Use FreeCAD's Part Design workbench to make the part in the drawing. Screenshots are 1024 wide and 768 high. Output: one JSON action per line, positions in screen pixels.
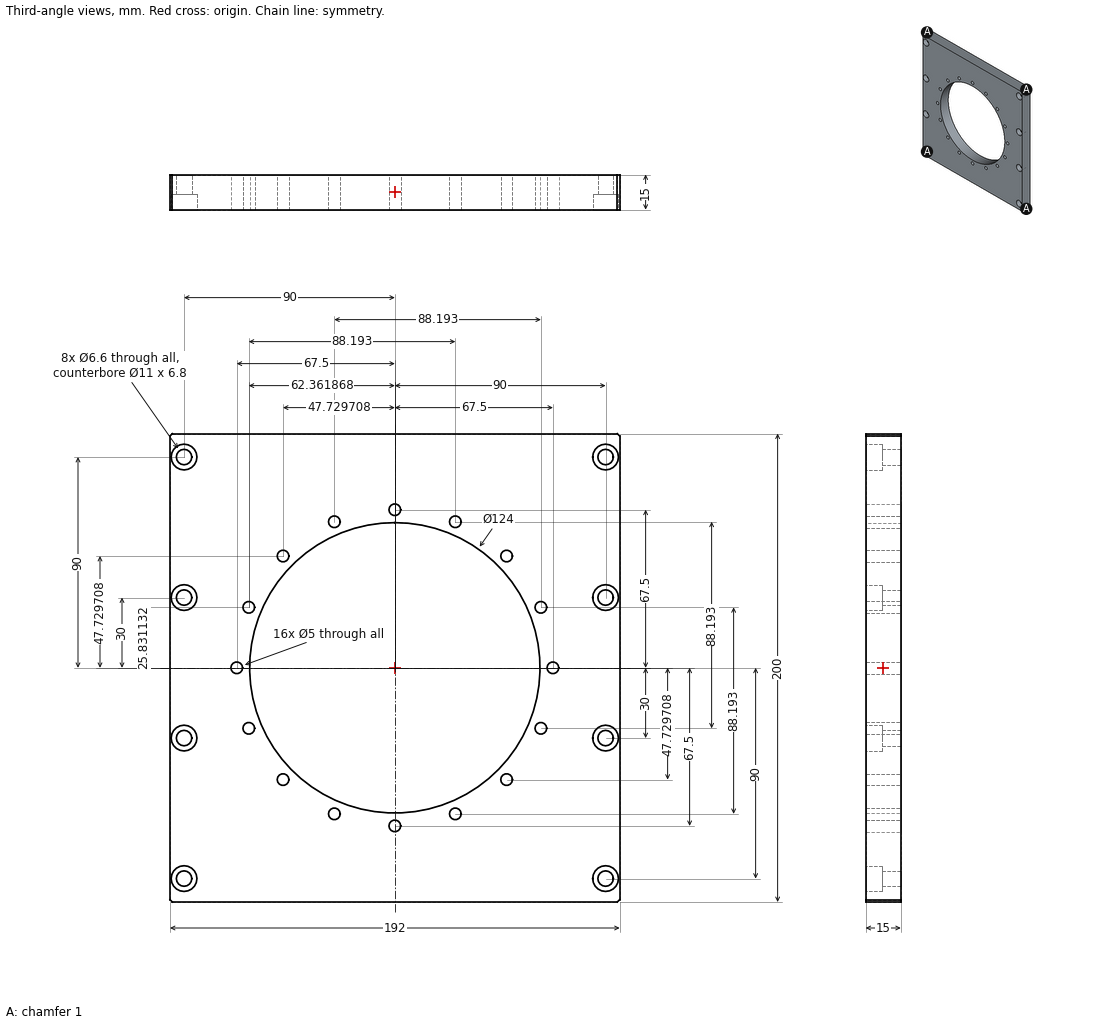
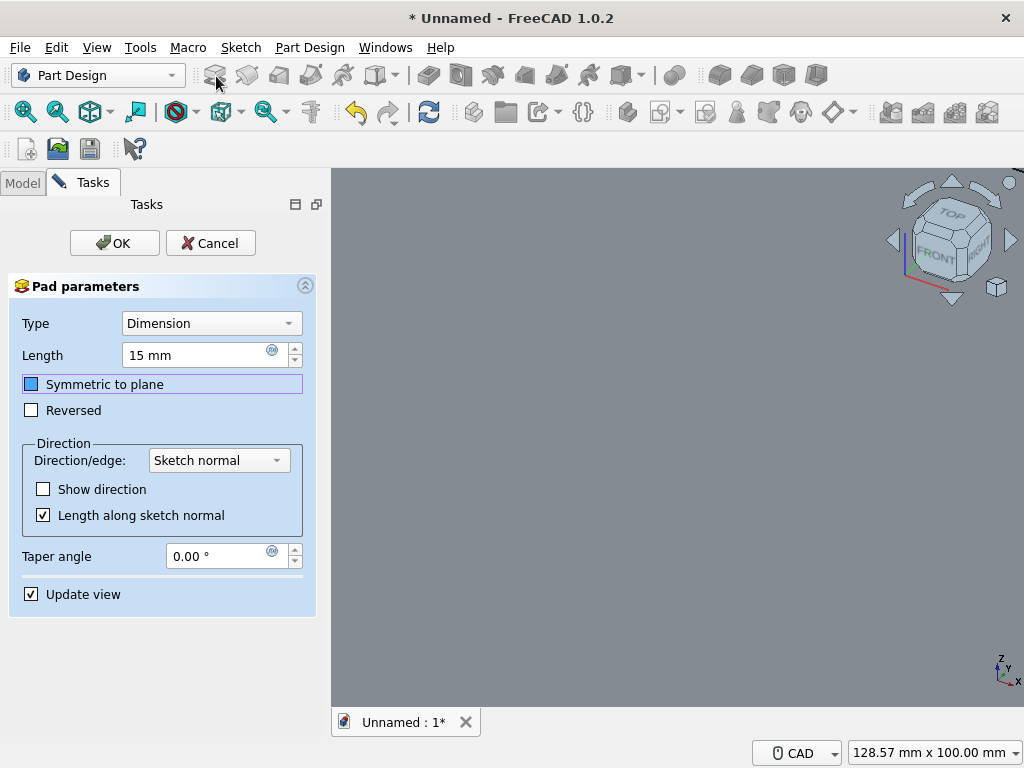
{"action": "left_click", "coordinate": [30, 384]}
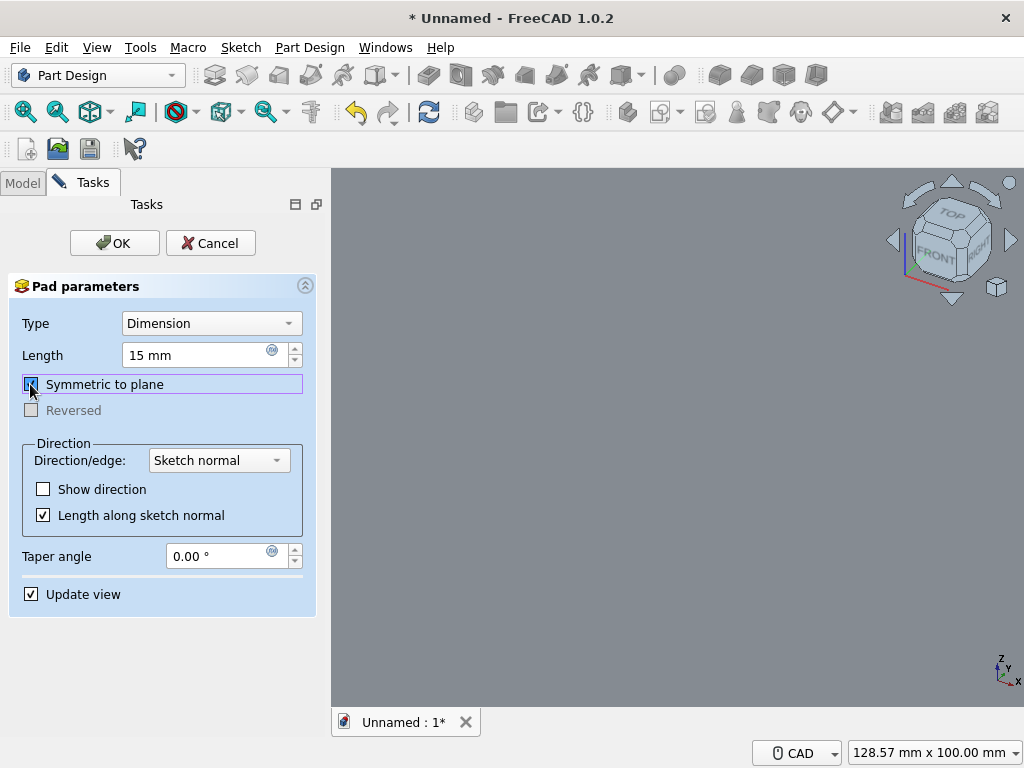
{"action": "left_click", "coordinate": [115, 243]}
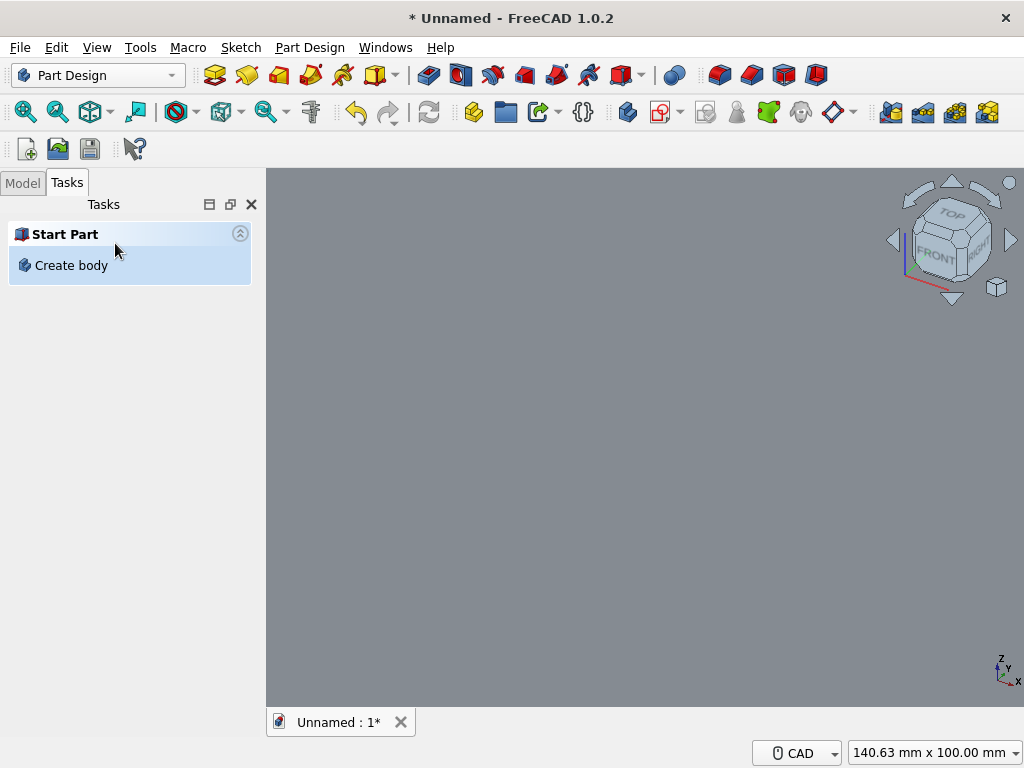
{"action": "left_click", "coordinate": [26, 112]}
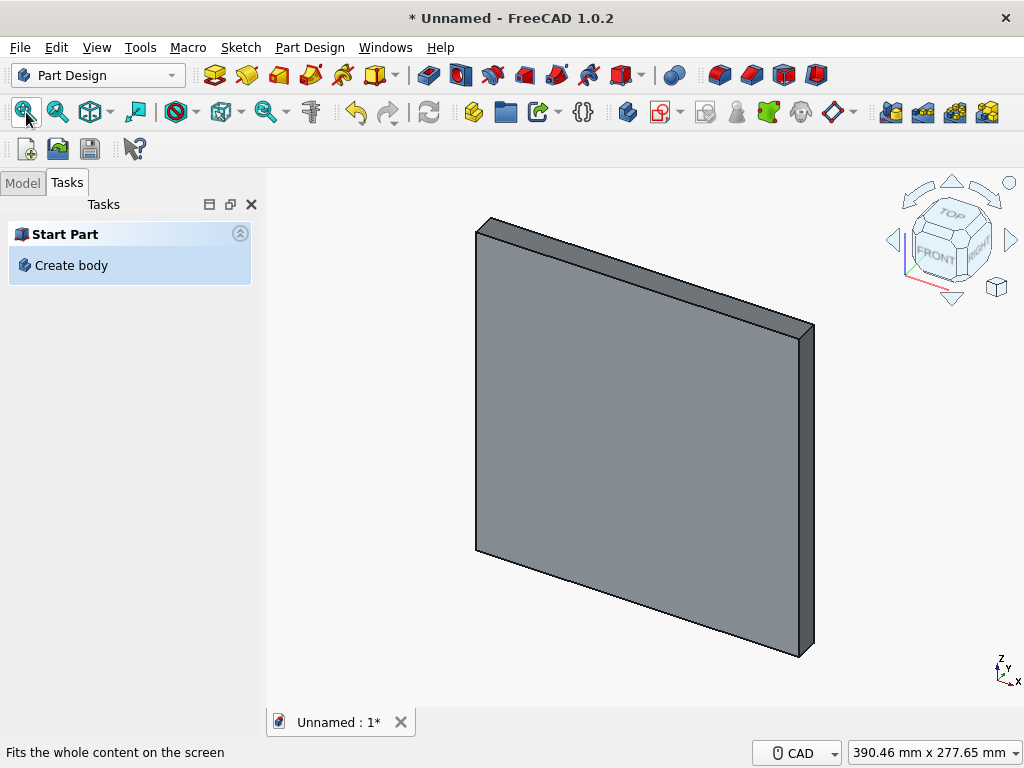
{"action": "left_click", "coordinate": [806, 331]}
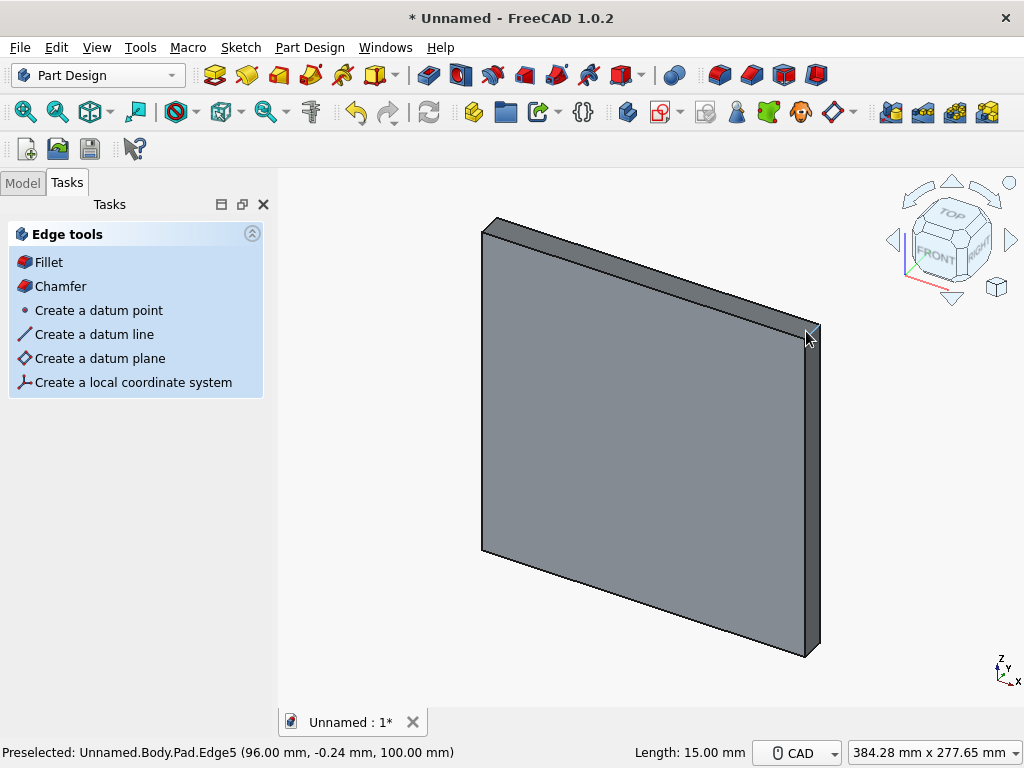
{"action": "key", "text": "0"}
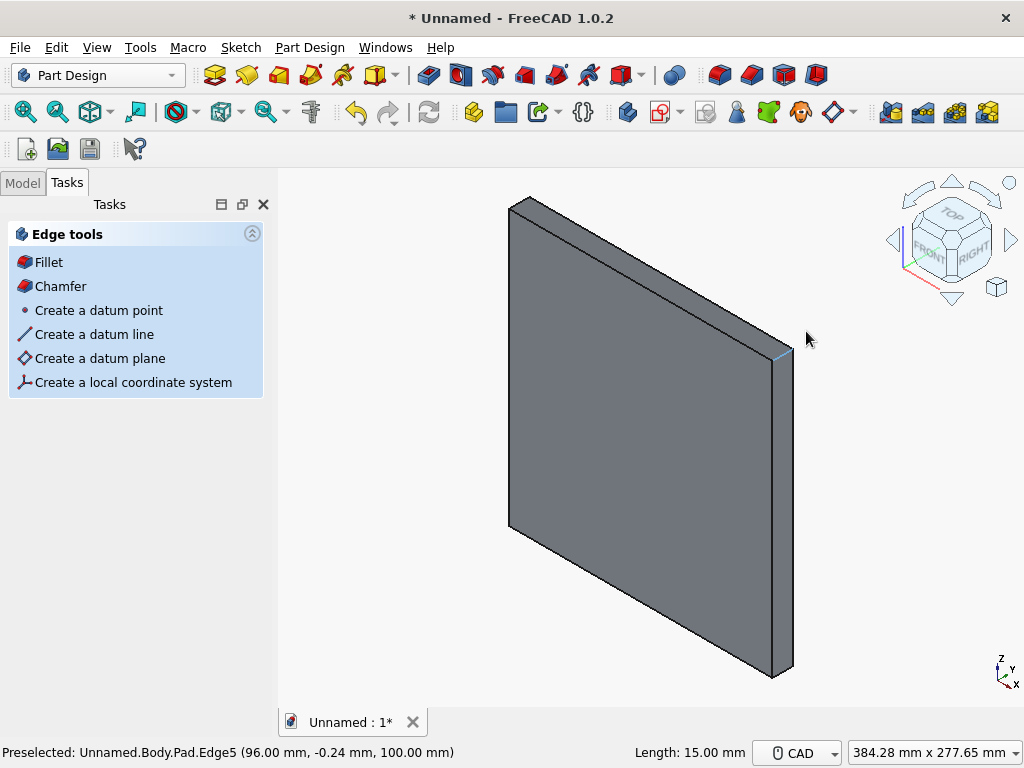
{"action": "key", "text": "2"}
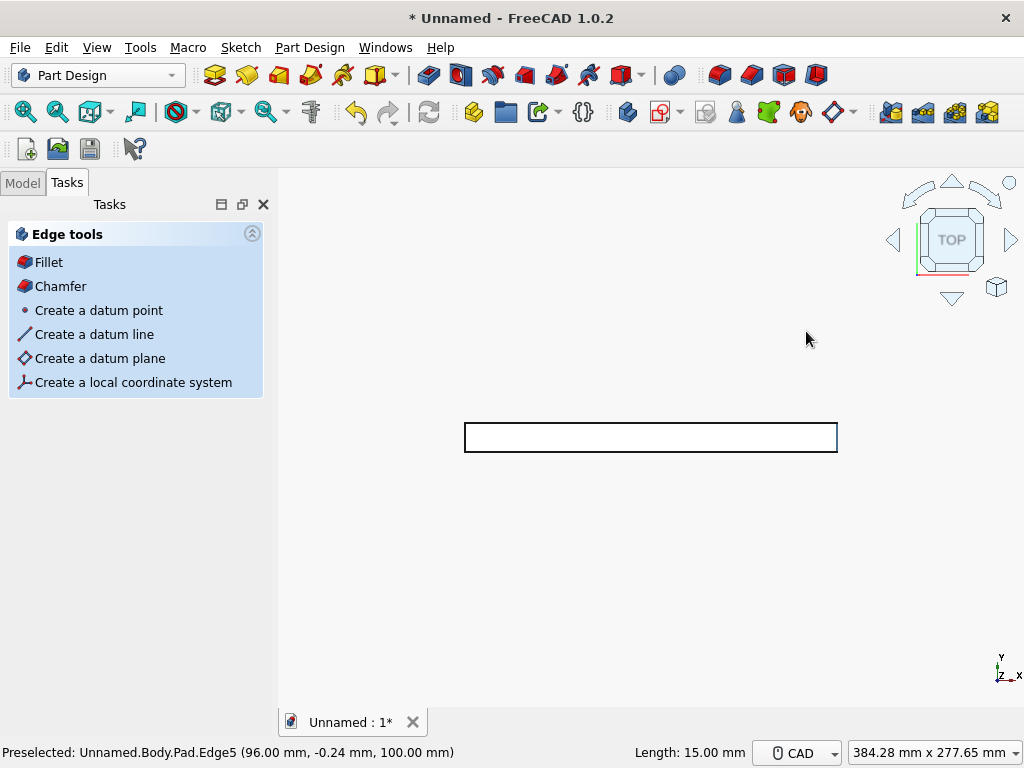
{"action": "left_click", "coordinate": [465, 436], "text": "ctrl"}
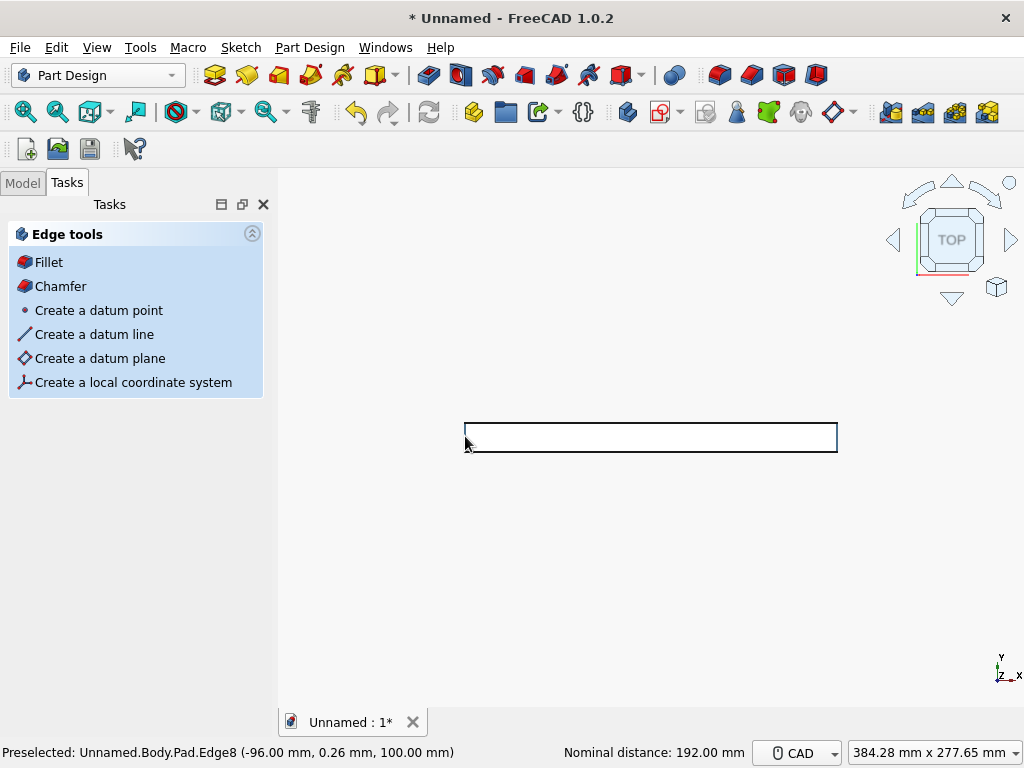
{"action": "key", "text": "1"}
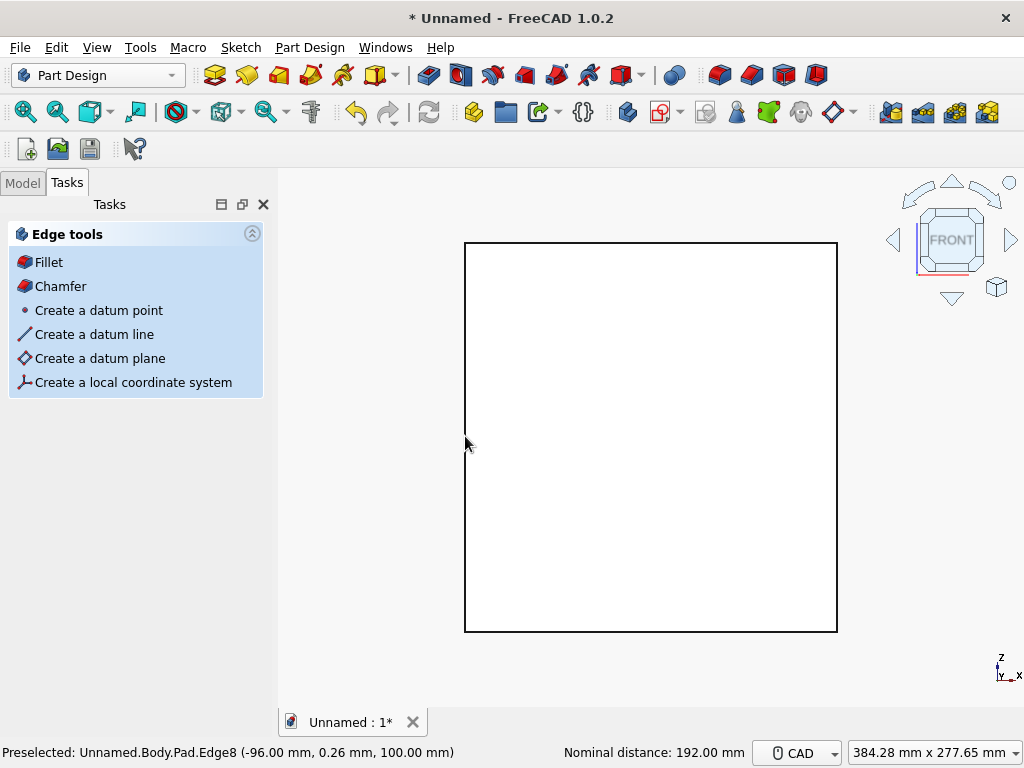
{"action": "key", "text": "3"}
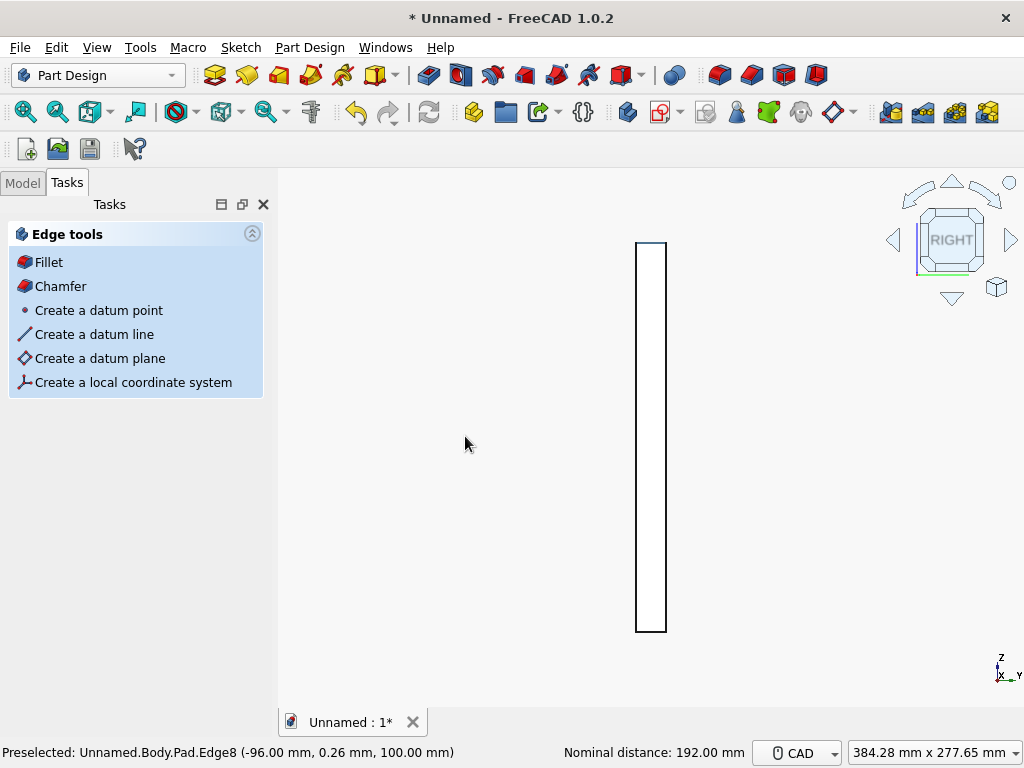
{"action": "left_click", "coordinate": [651, 631], "text": "ctrl"}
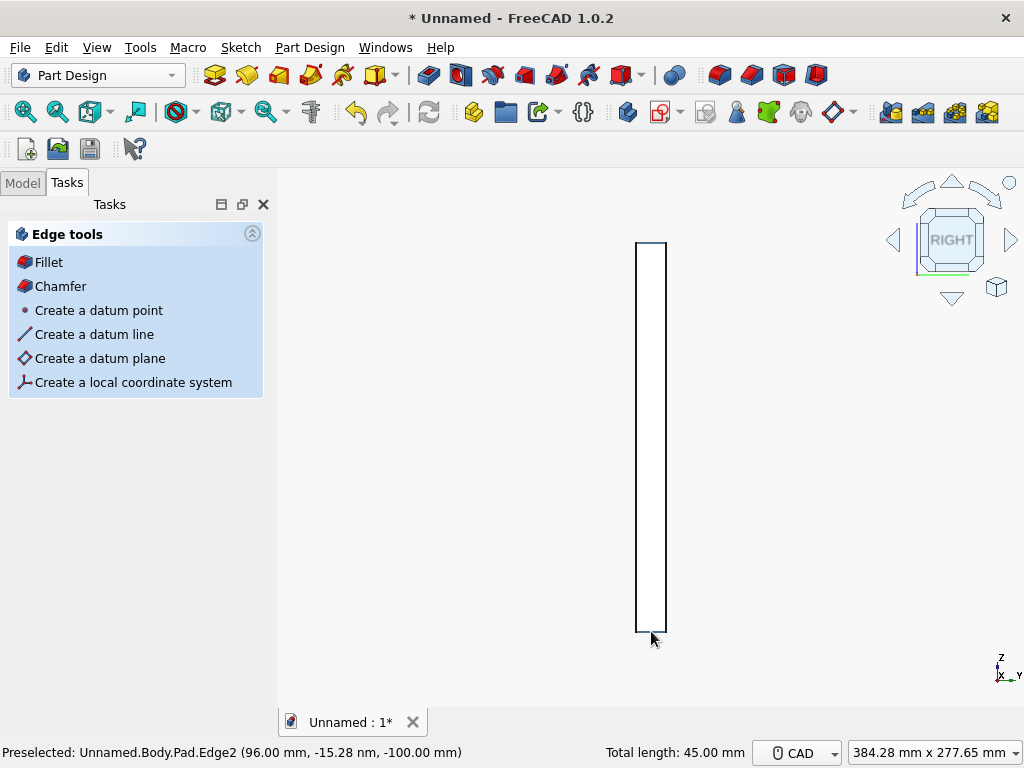
{"action": "key", "text": "5"}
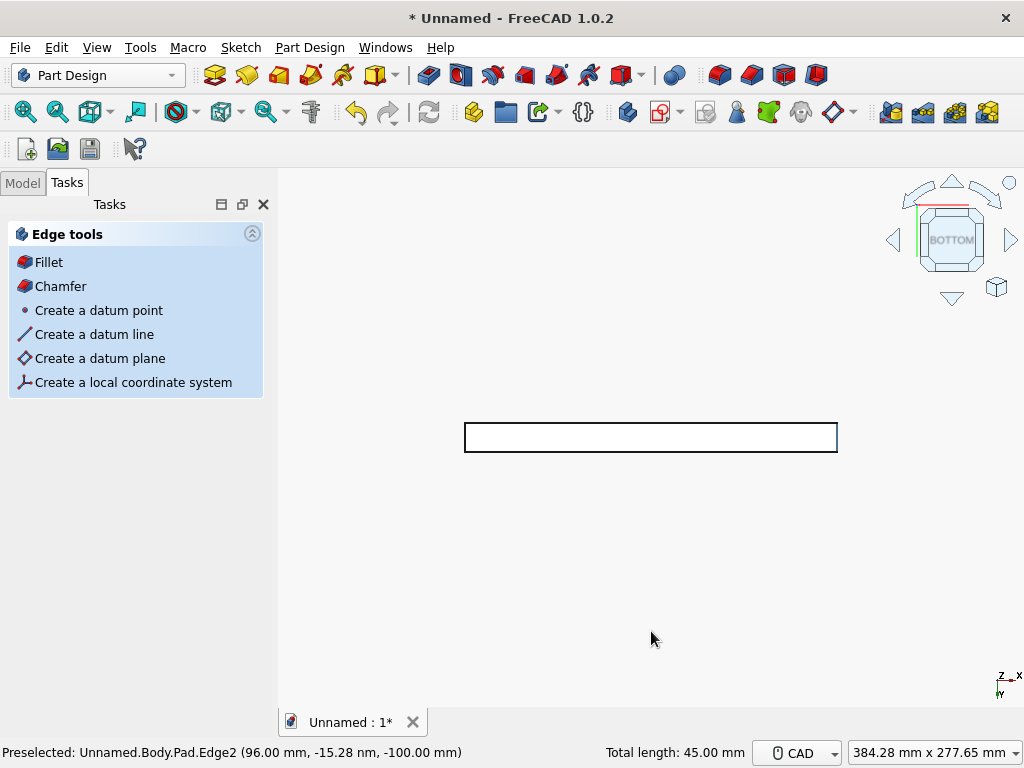
{"action": "left_click", "coordinate": [465, 437], "text": "ctrl"}